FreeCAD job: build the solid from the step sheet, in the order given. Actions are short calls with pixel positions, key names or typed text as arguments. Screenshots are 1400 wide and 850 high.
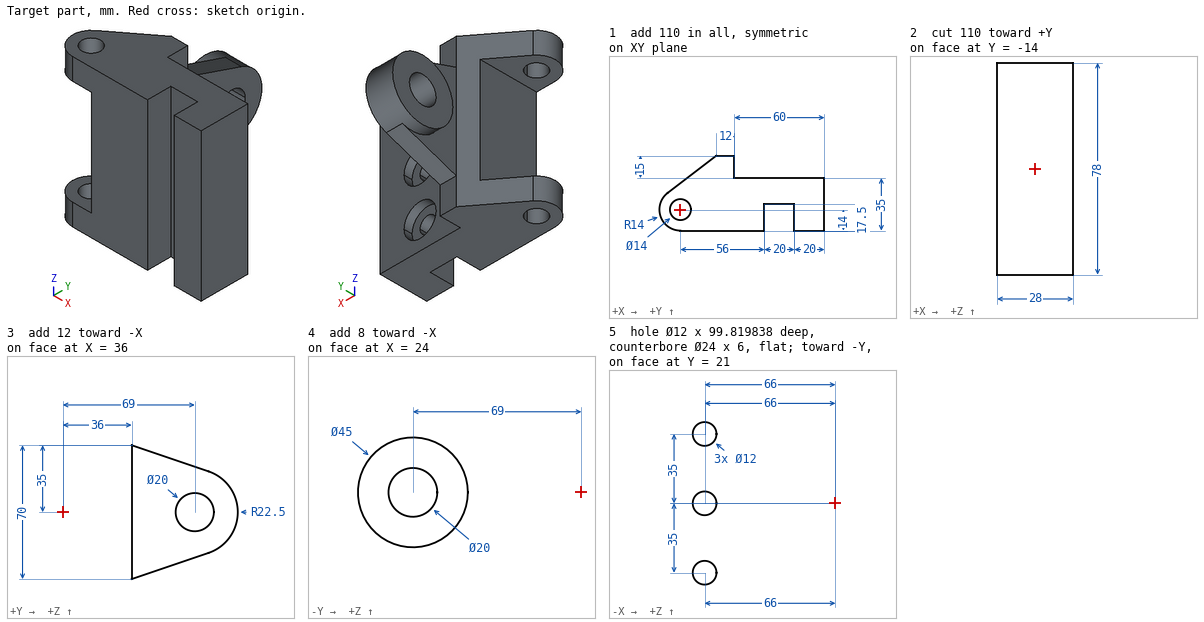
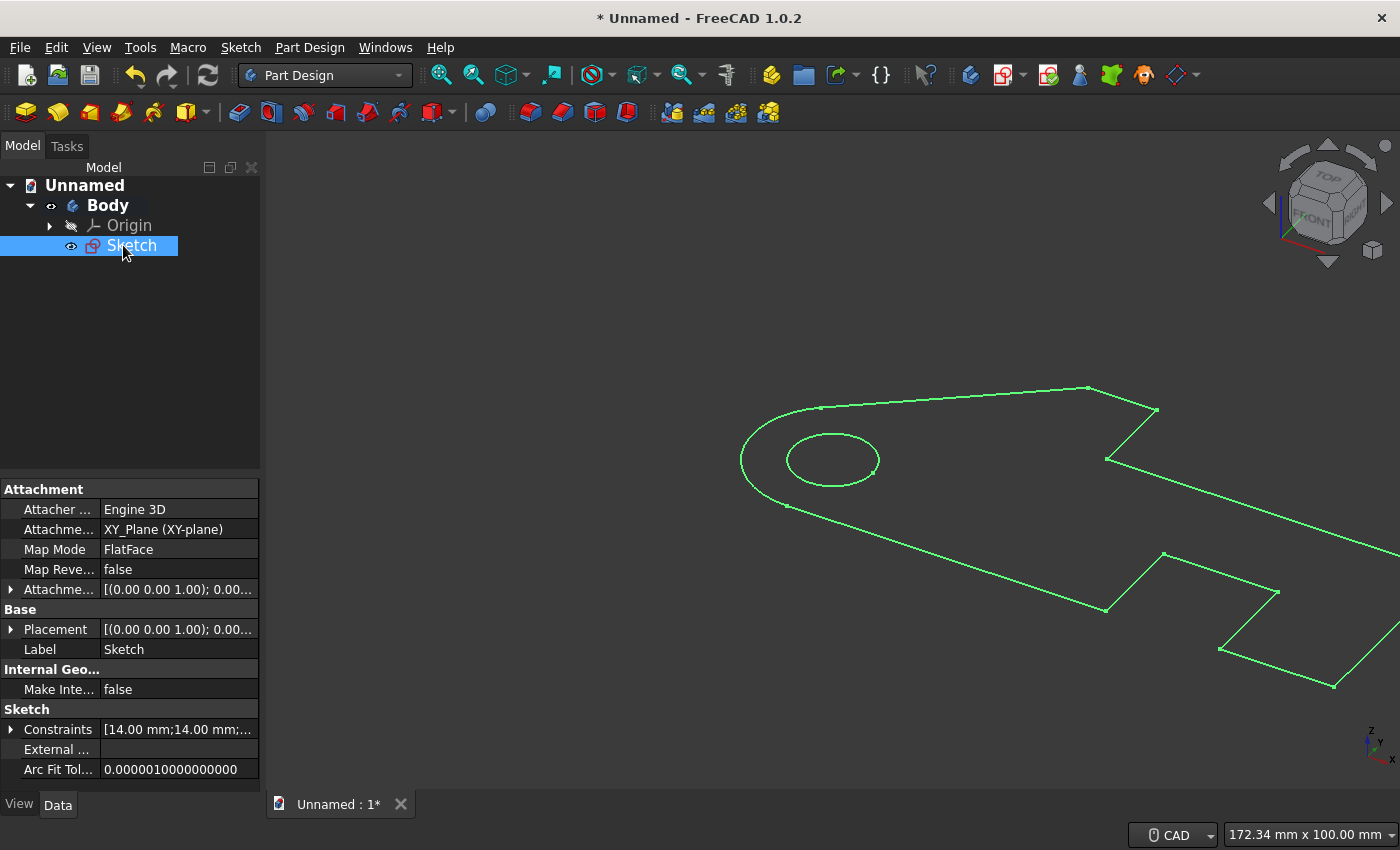
click(26, 112)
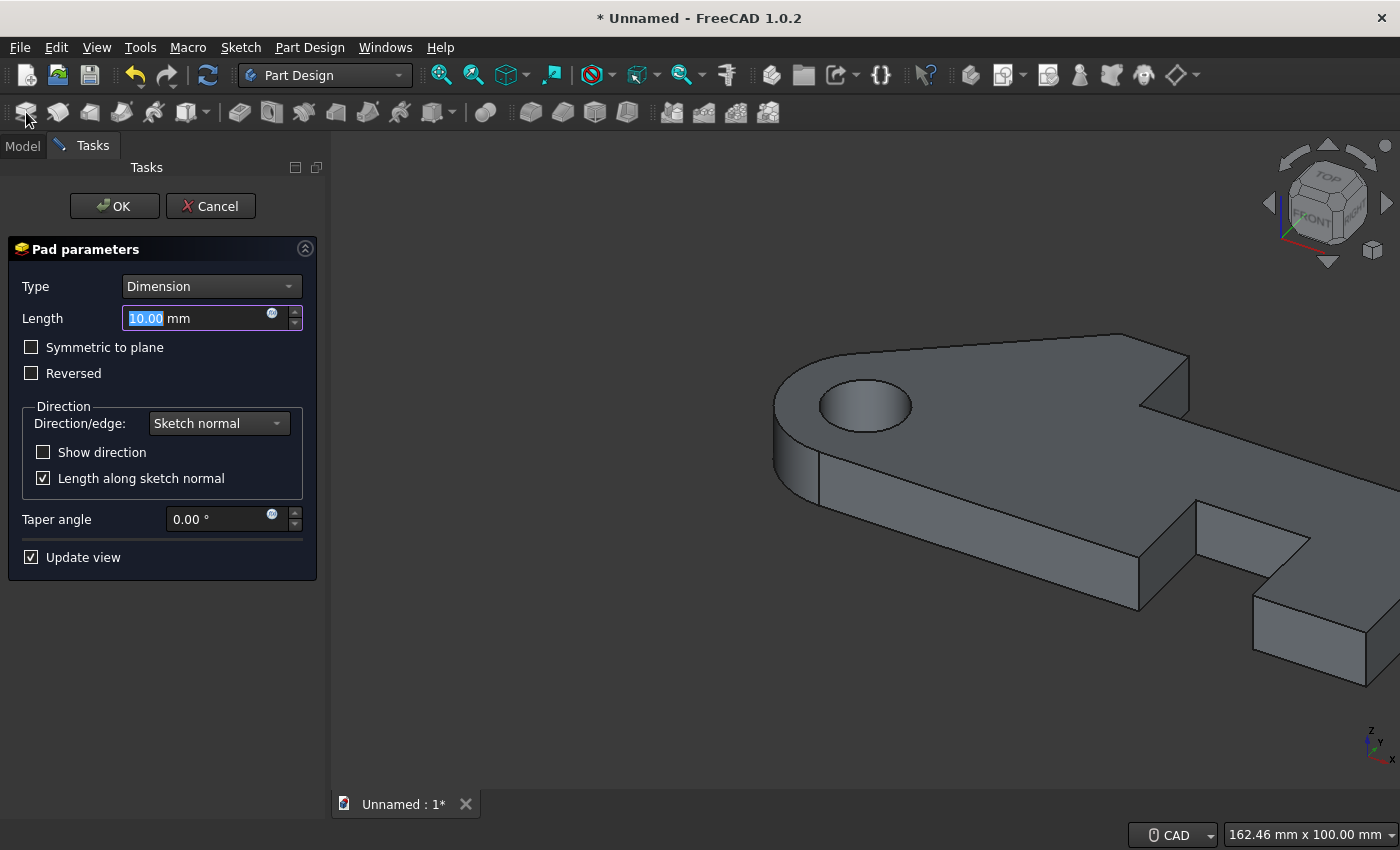
text(110)
key(Tab)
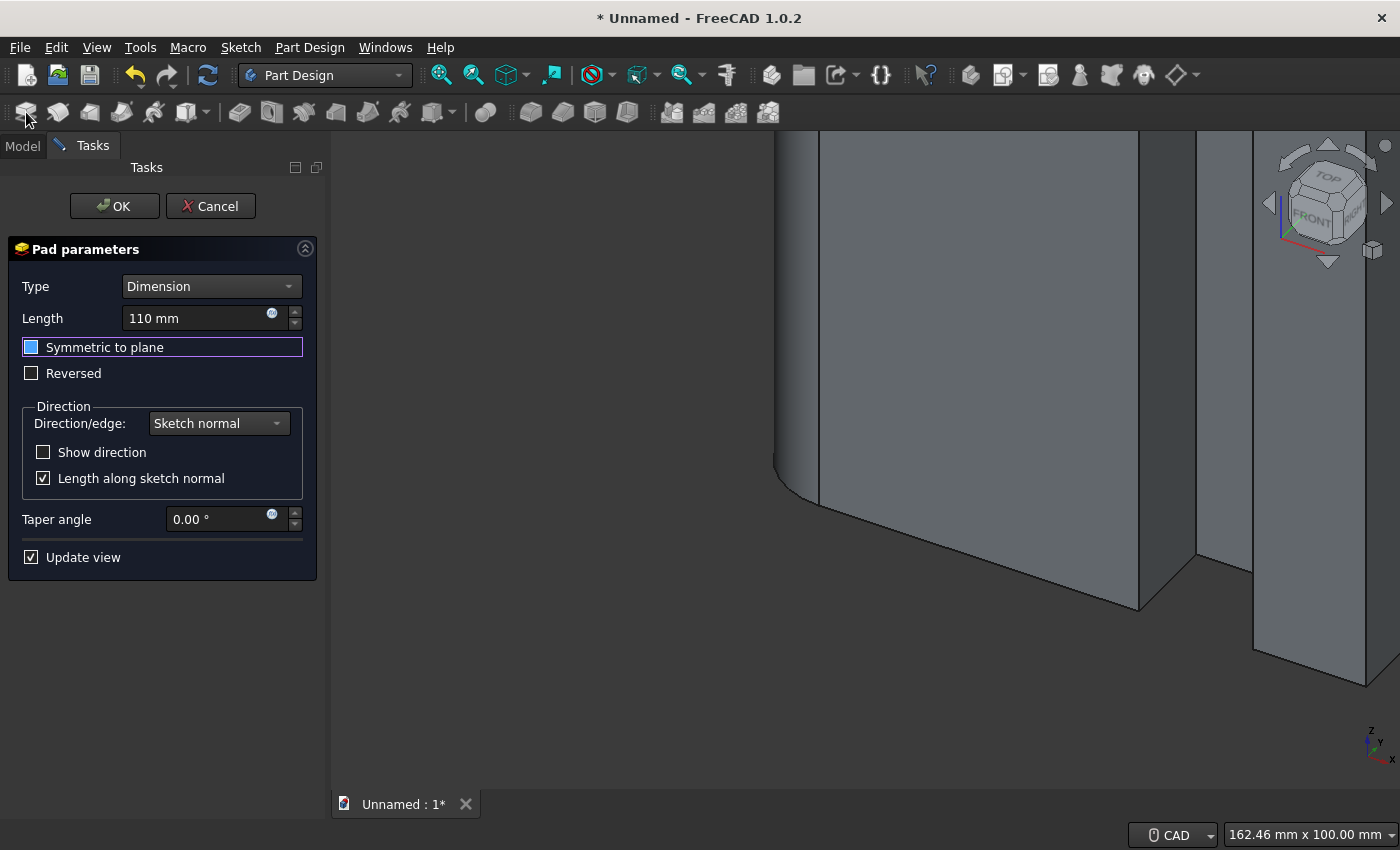
click(30, 347)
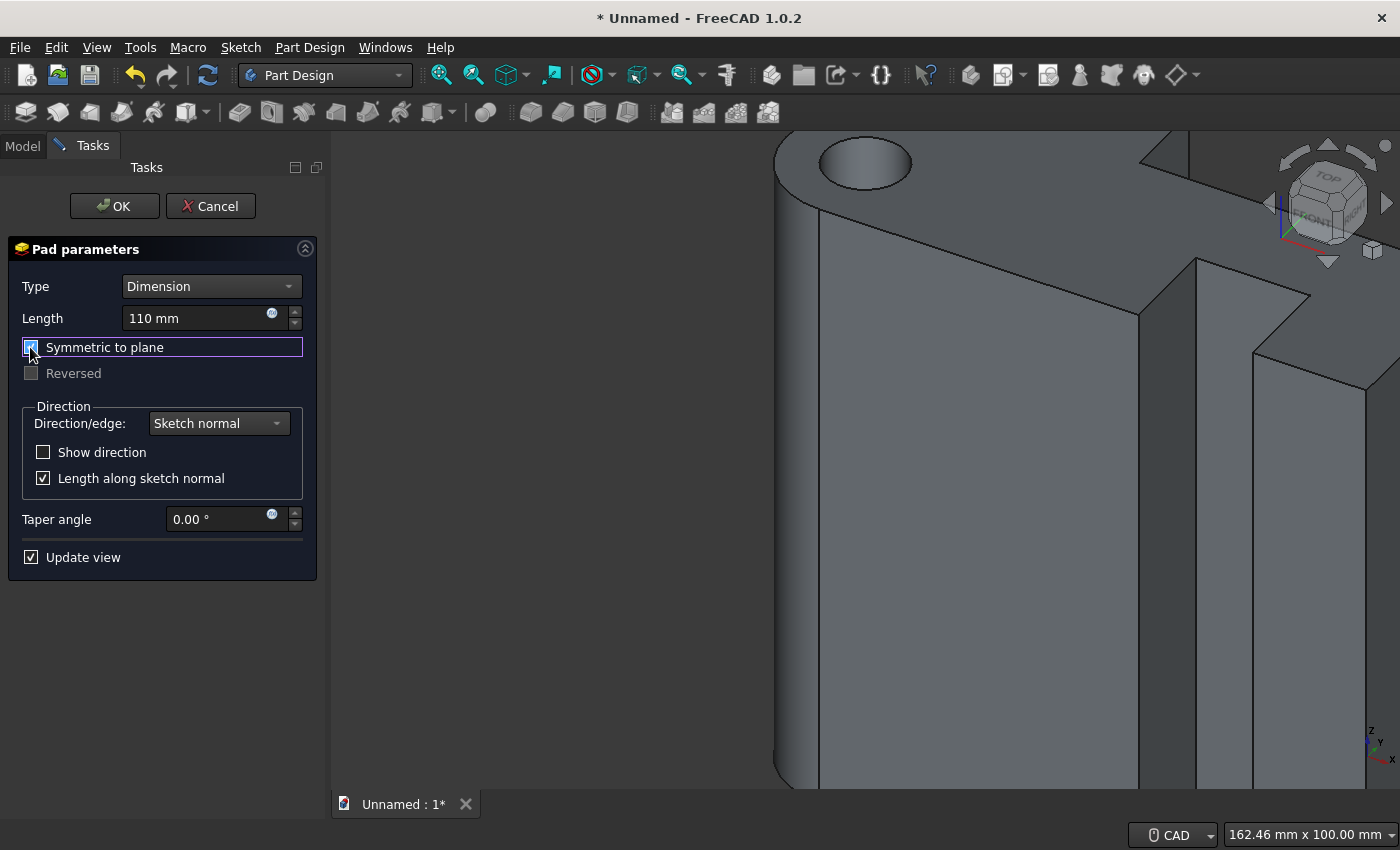
click(115, 206)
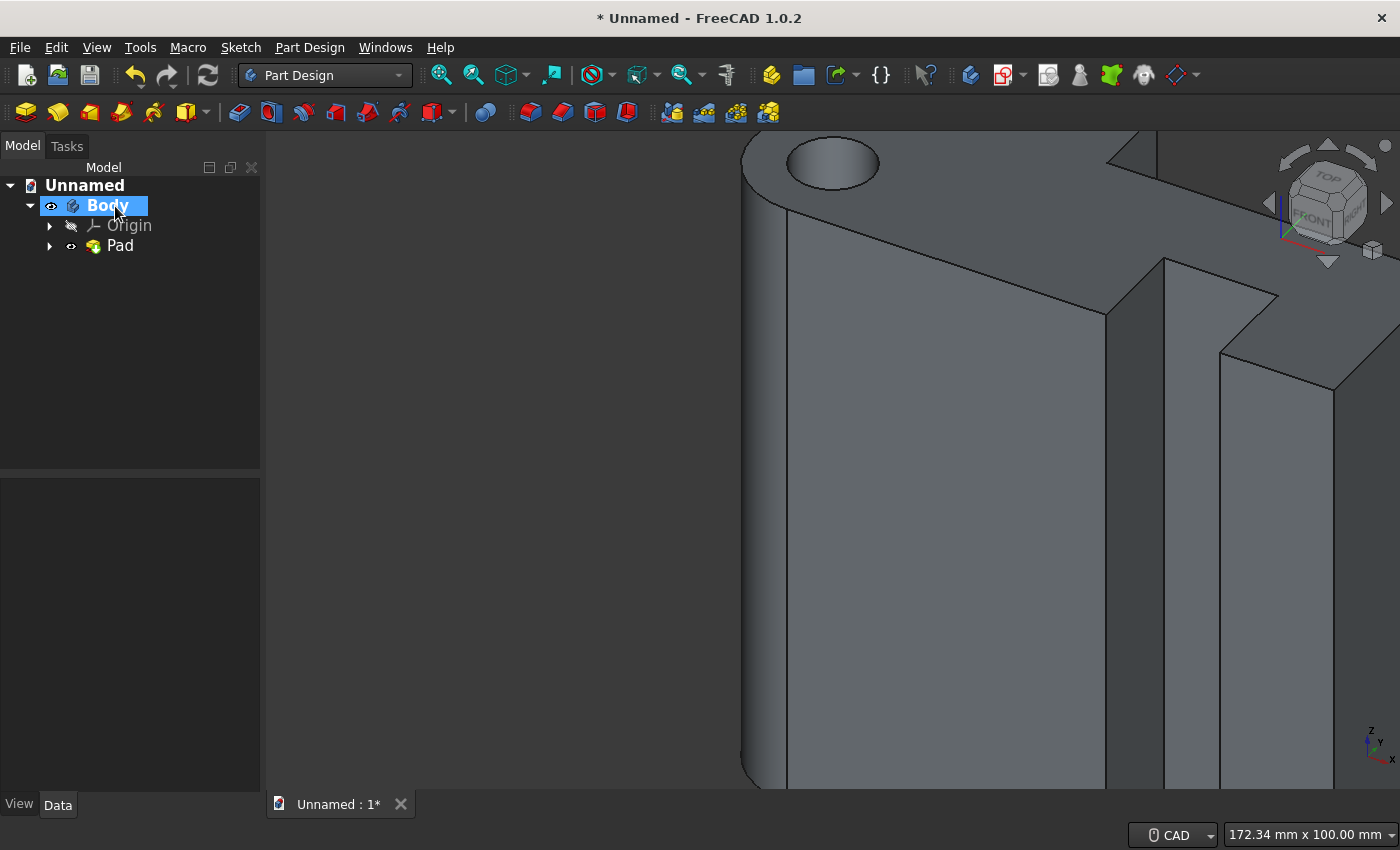
click(442, 76)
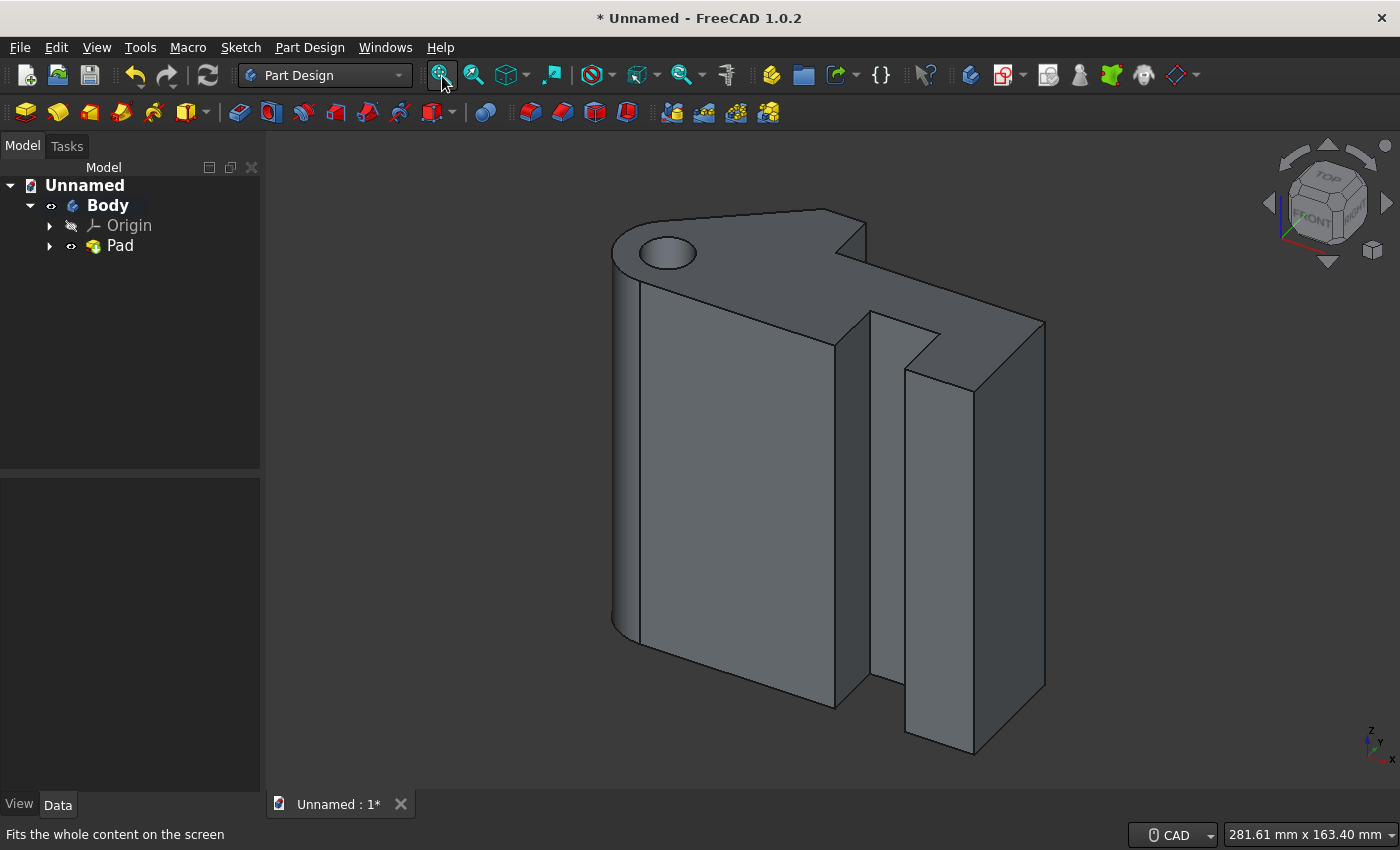
click(737, 442)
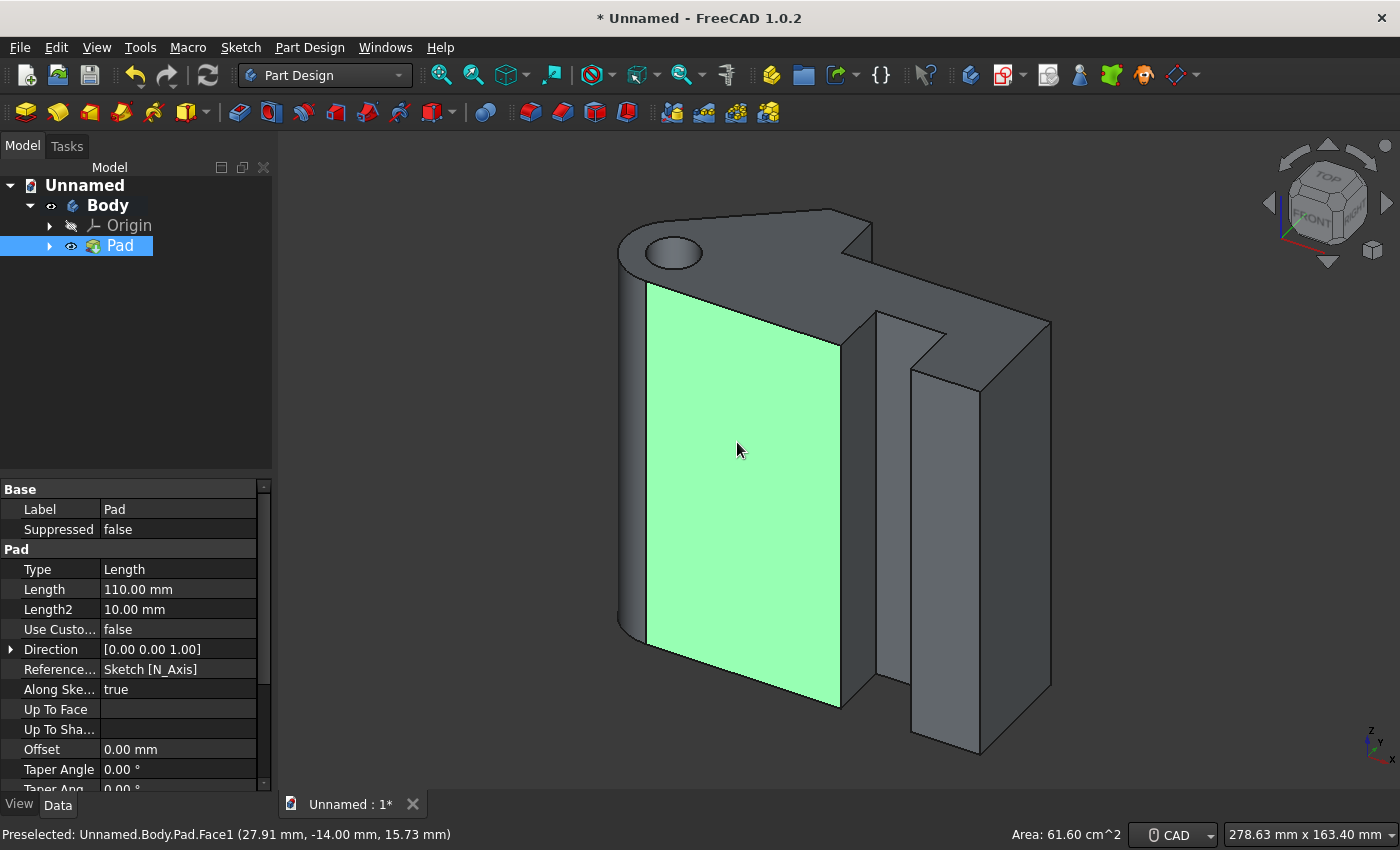
click(1004, 76)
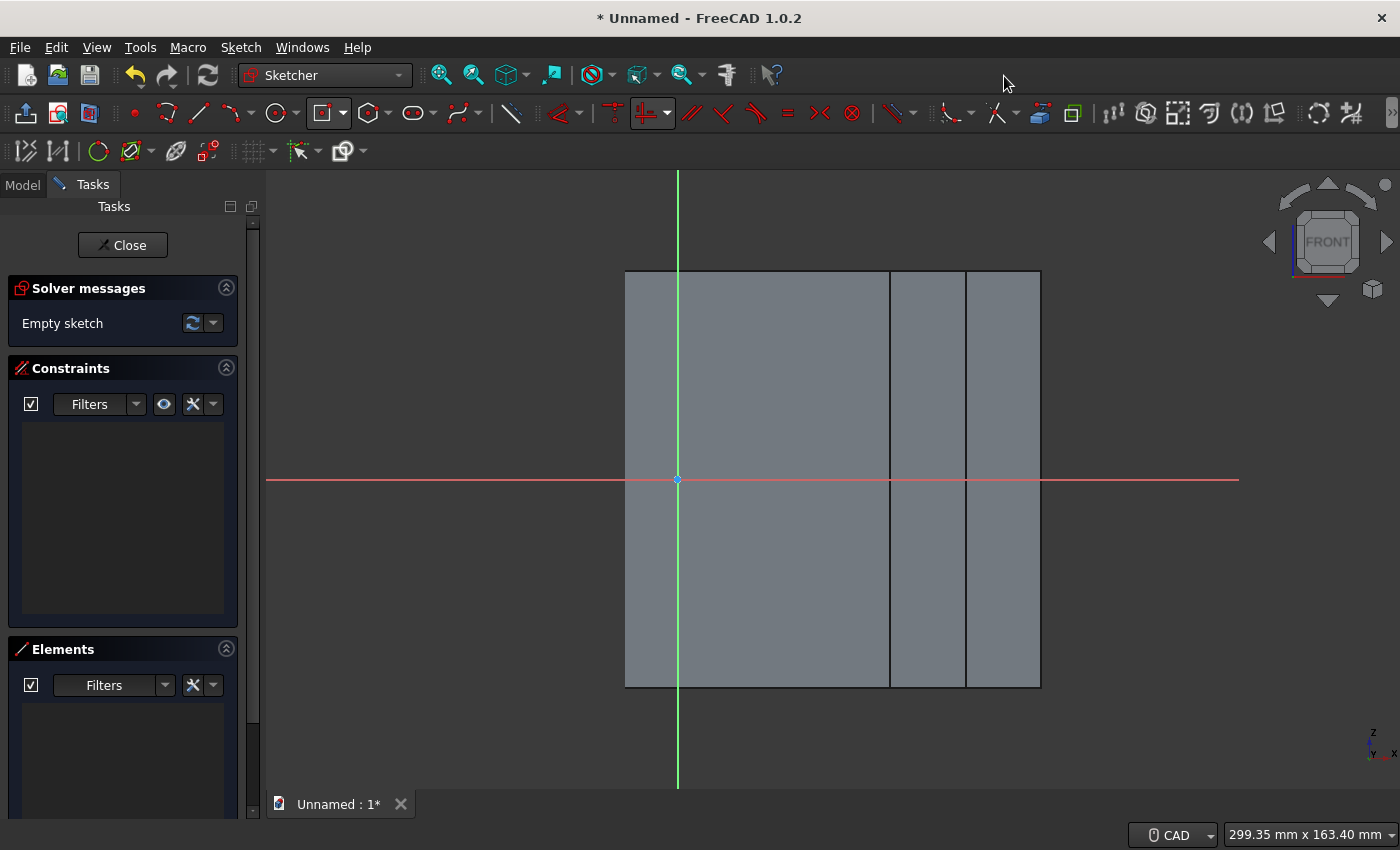
key(g)
key(v)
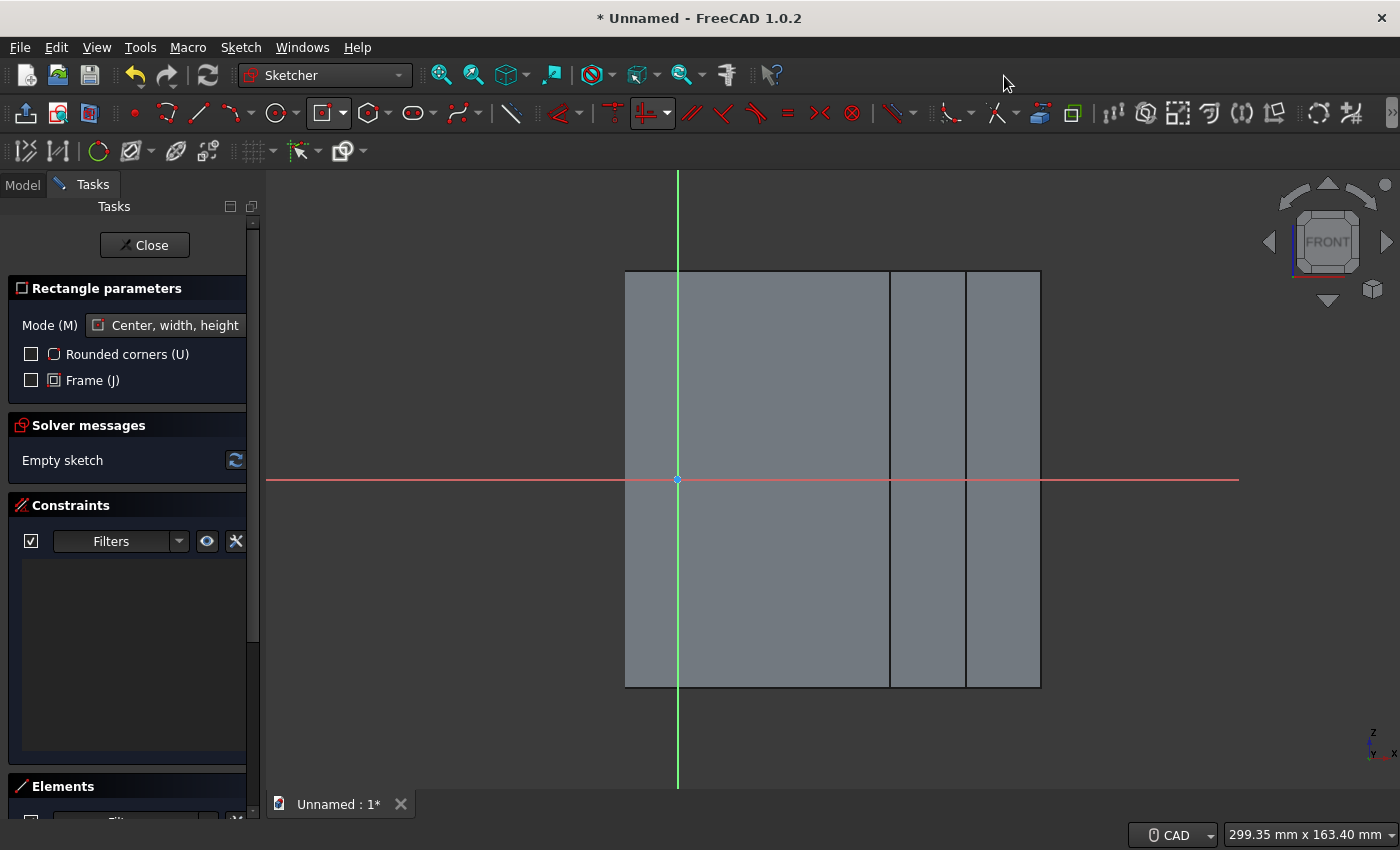
click(678, 480)
click(731, 332)
key(Escape)